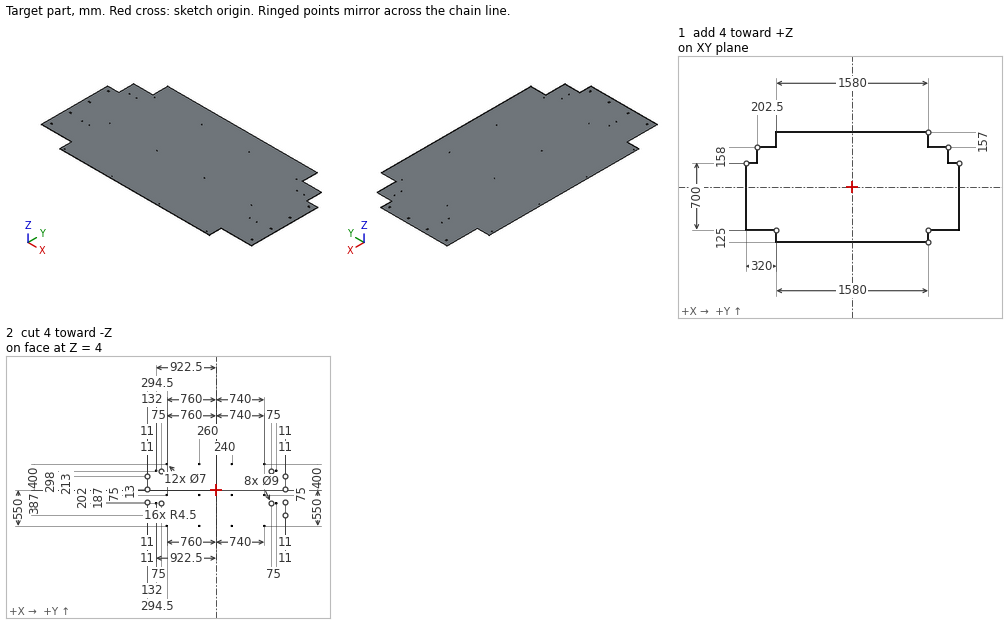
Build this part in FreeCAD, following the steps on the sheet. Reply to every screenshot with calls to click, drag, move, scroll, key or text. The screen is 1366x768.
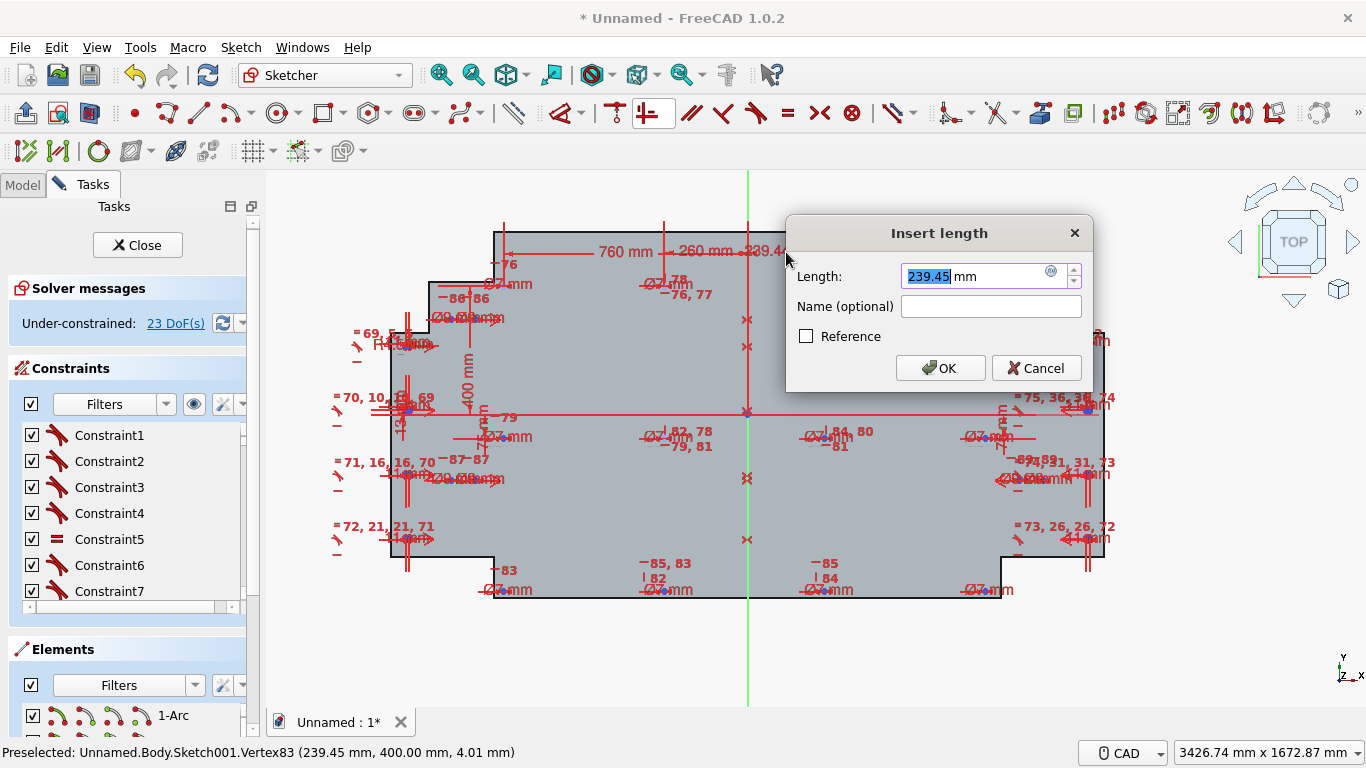
text(240)
key(Return)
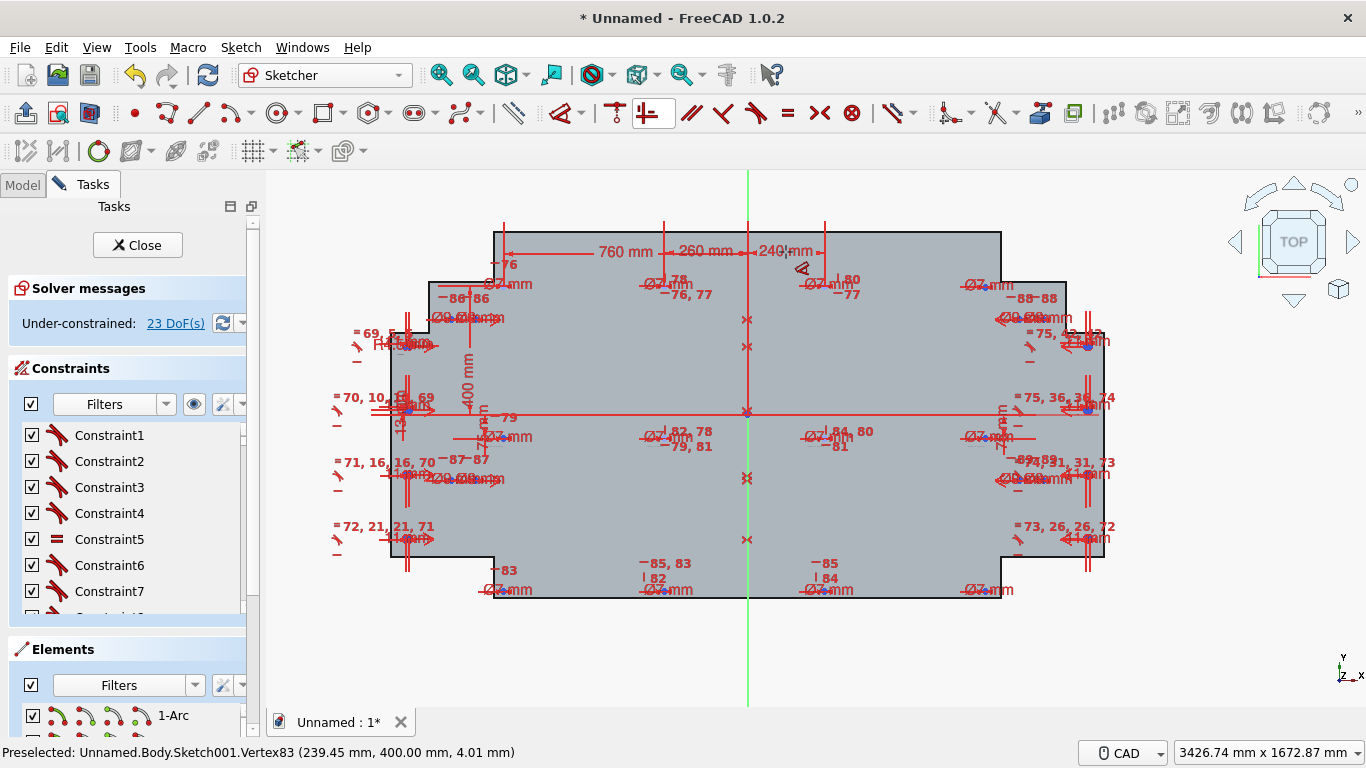
click(985, 287)
click(866, 253)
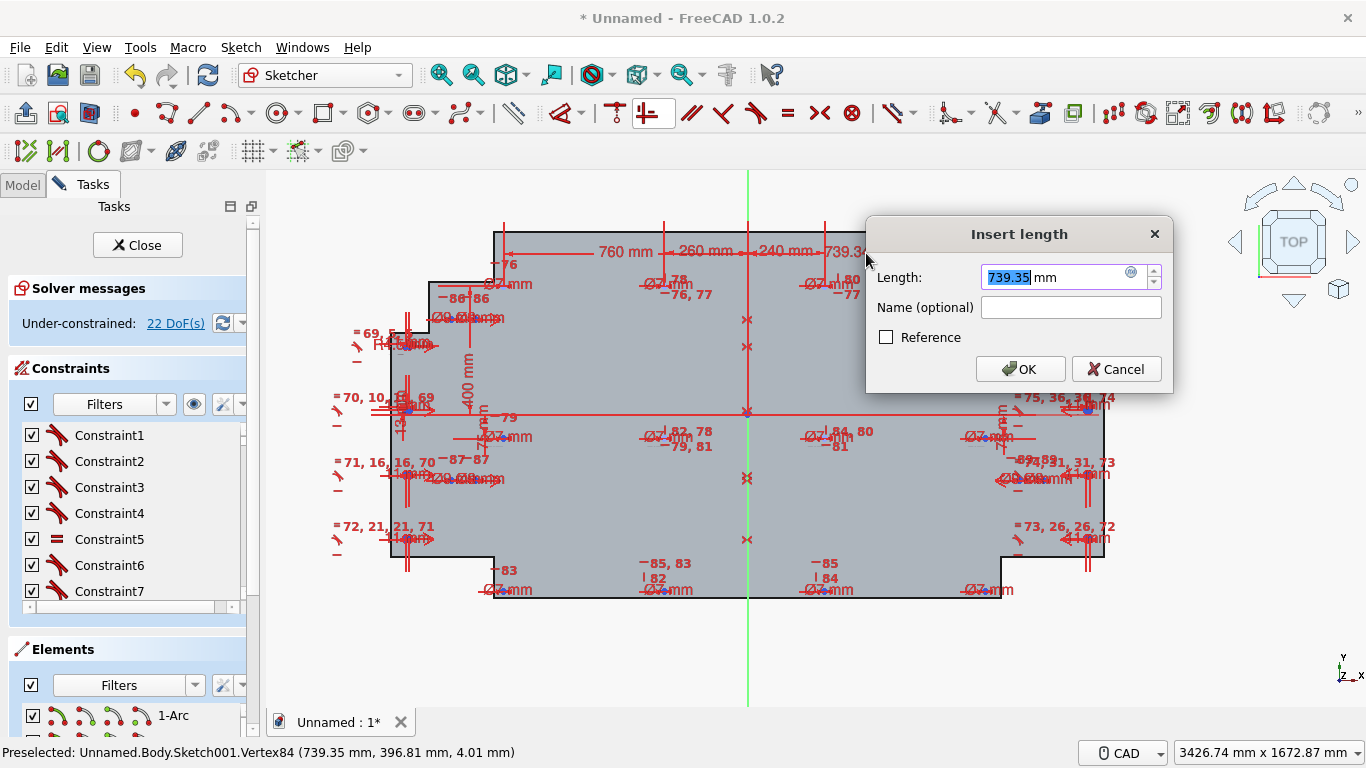
text(740)
key(Return)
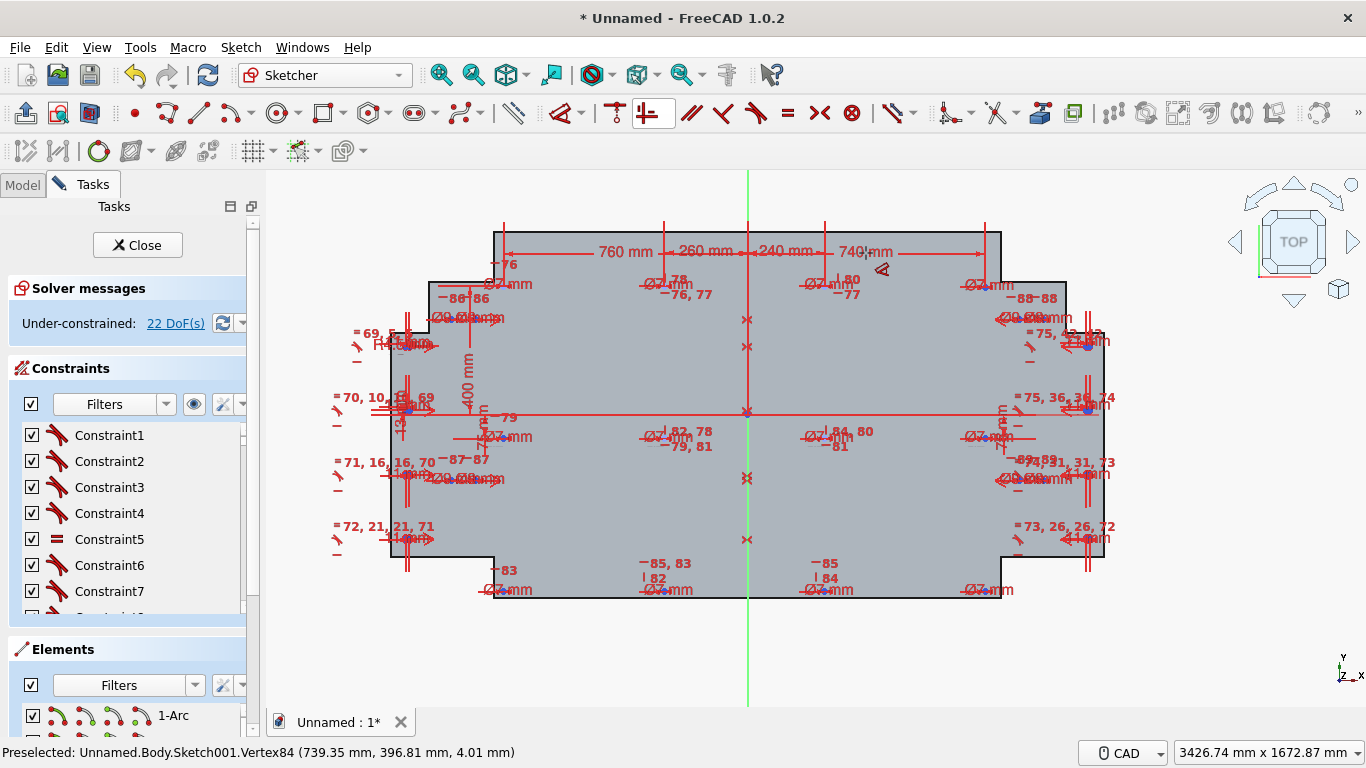
click(985, 287)
click(1019, 380)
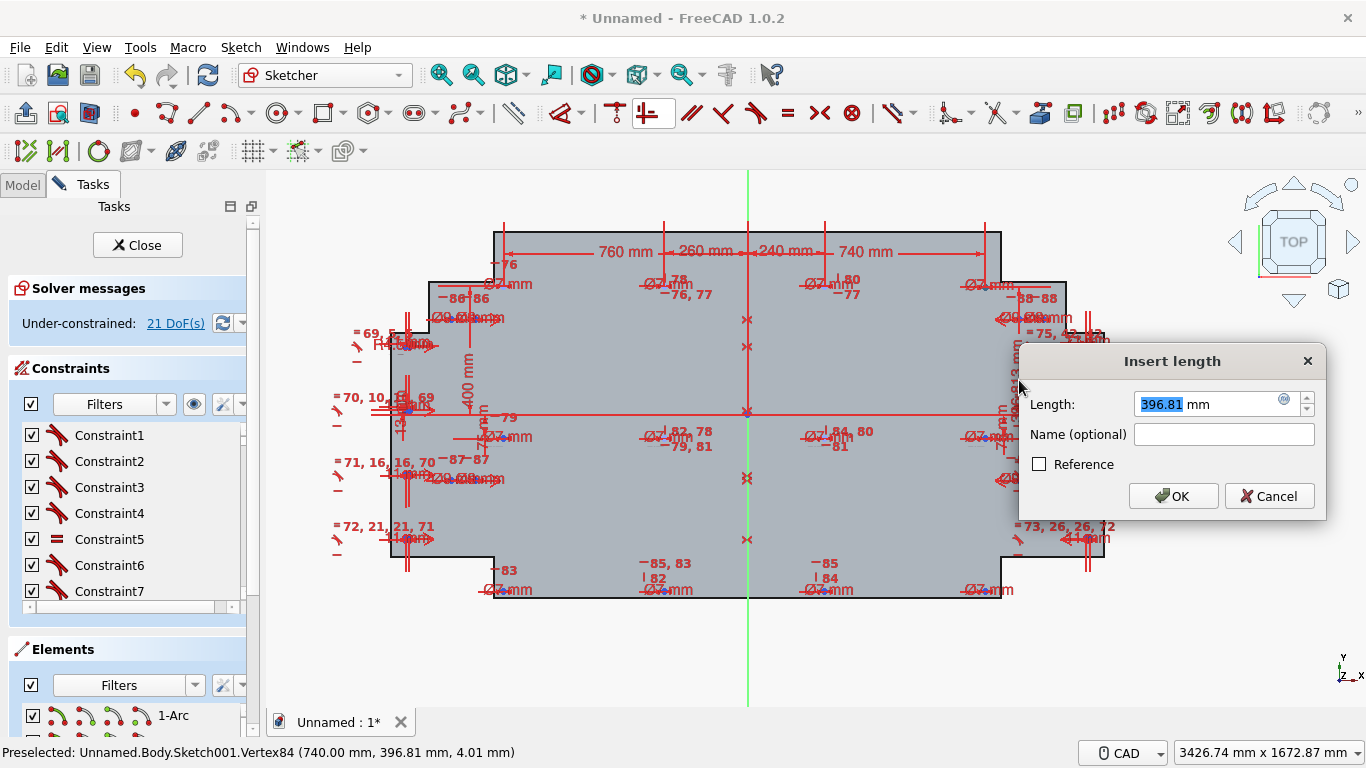
text(400)
key(Return)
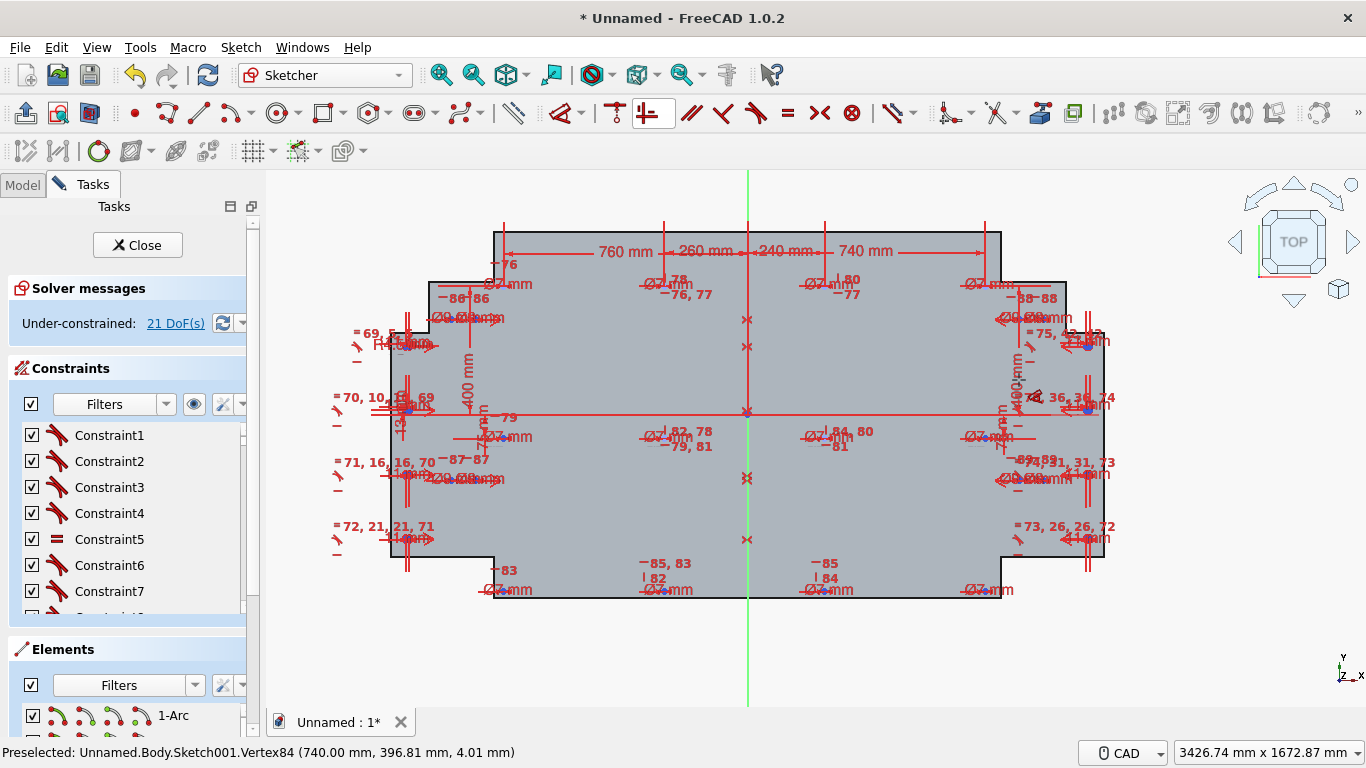
click(504, 439)
click(626, 381)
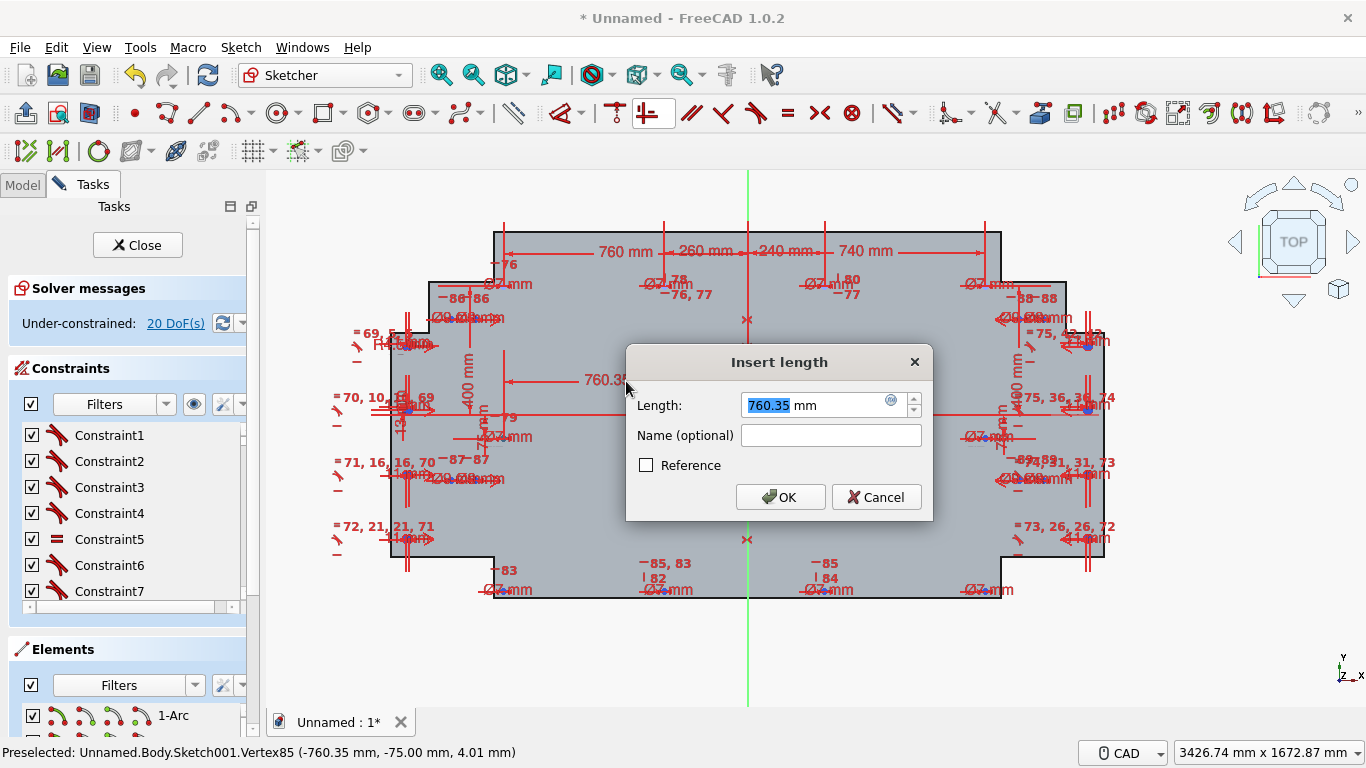
text(760)
key(Return)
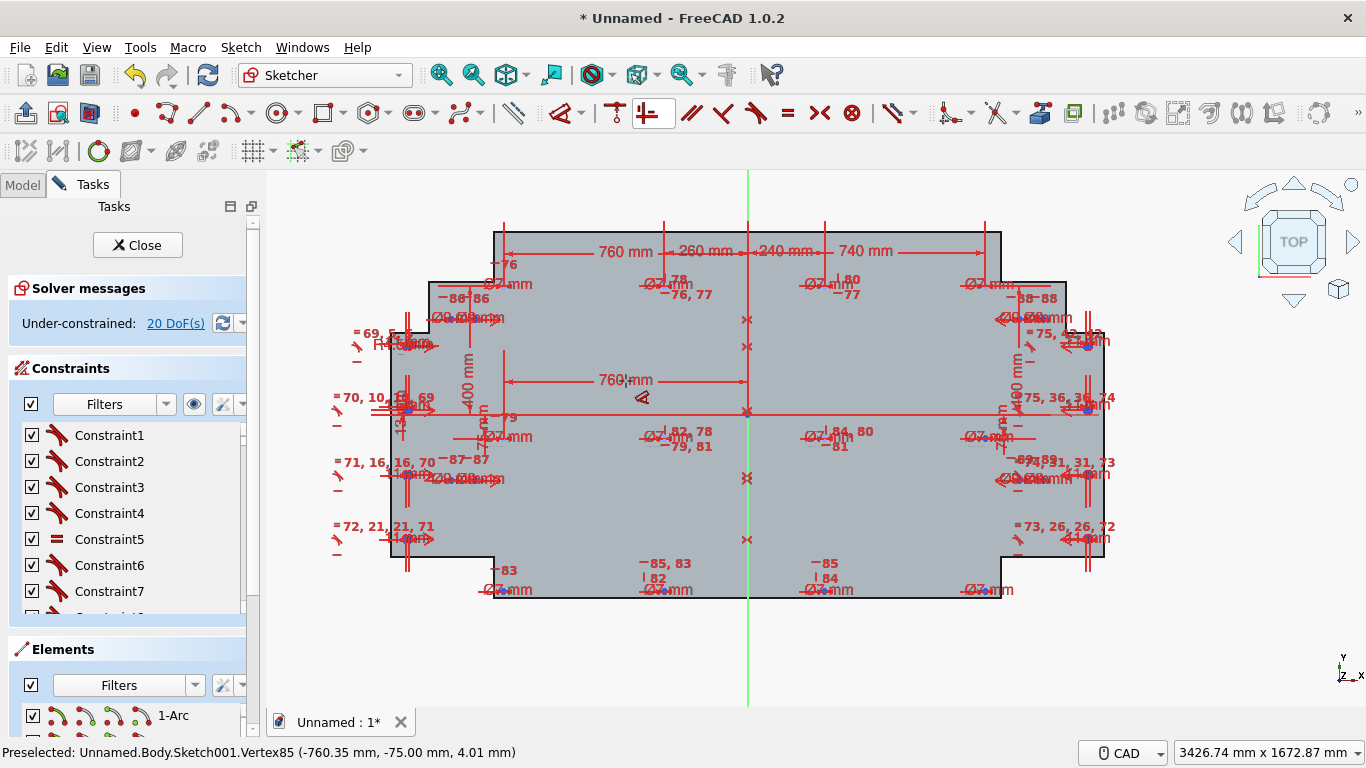
click(985, 439)
click(866, 381)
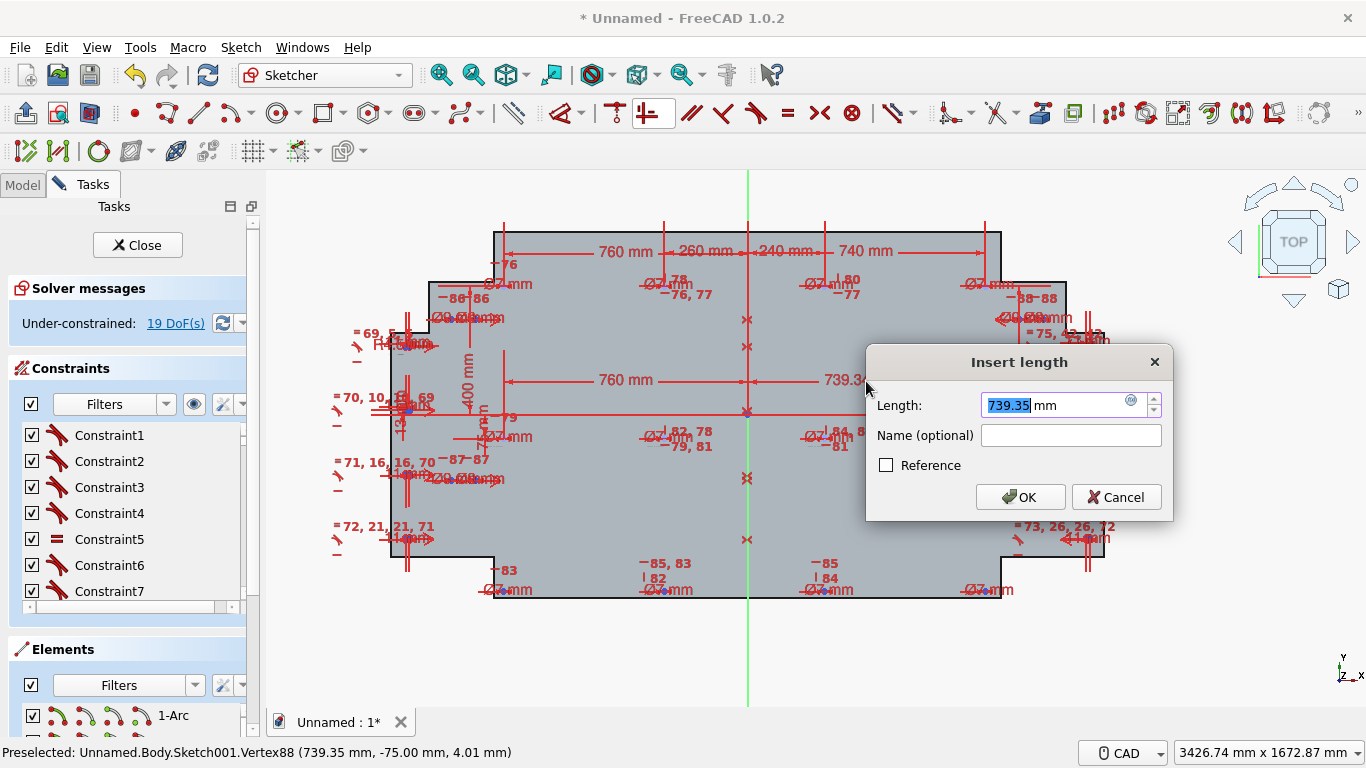
text(740)
key(Return)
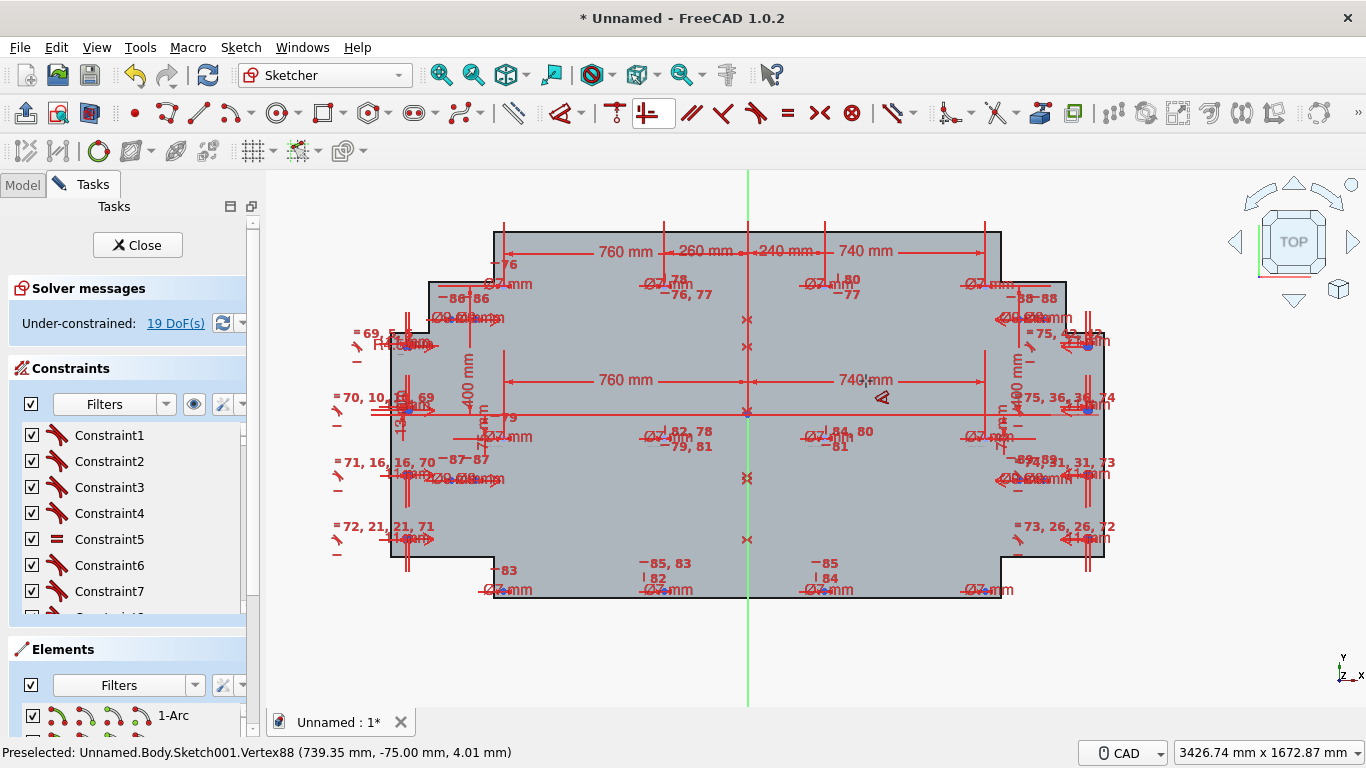
click(504, 592)
click(626, 626)